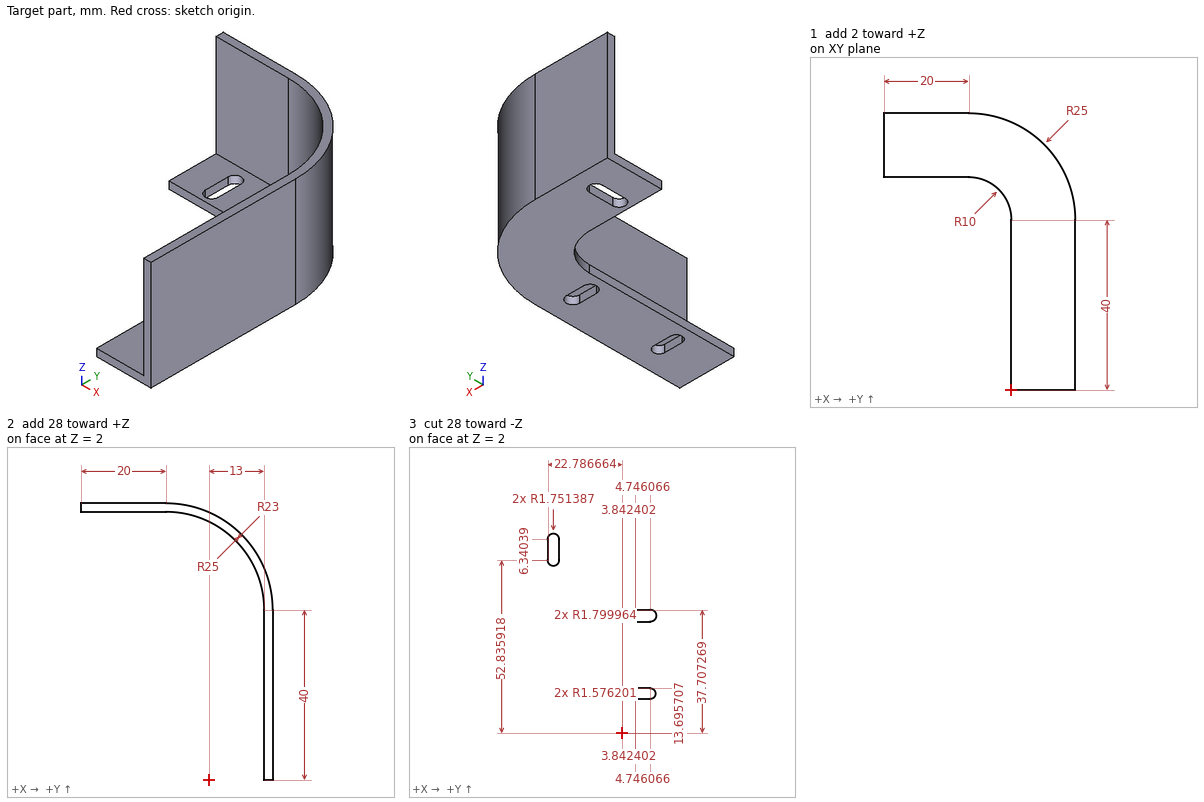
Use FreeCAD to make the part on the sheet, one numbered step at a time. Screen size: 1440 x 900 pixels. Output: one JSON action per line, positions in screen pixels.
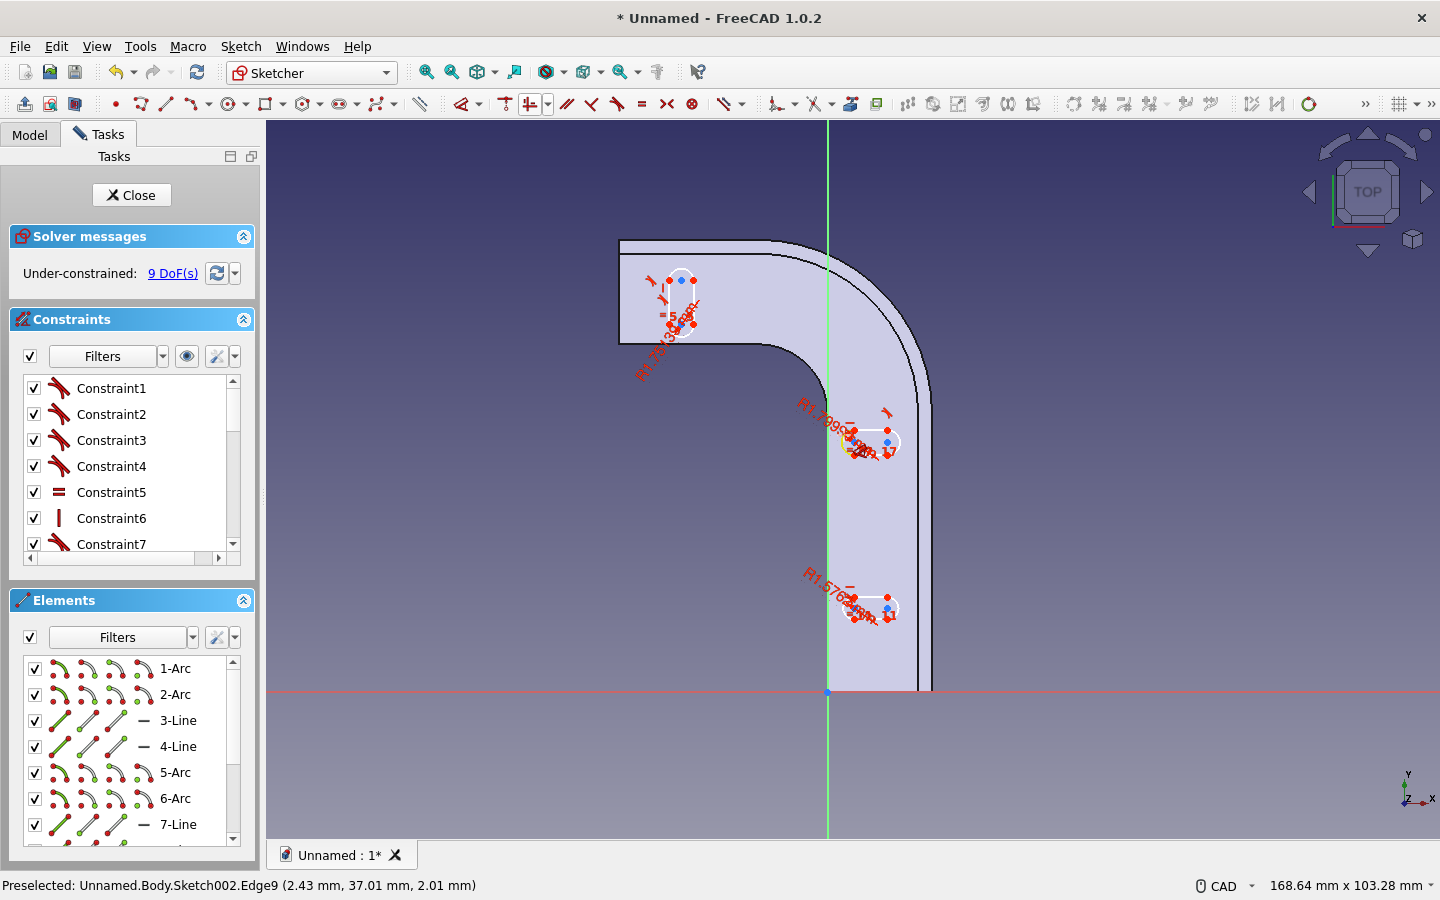
{"action": "left_click", "coordinate": [669, 312]}
{"action": "left_click", "coordinate": [635, 303]}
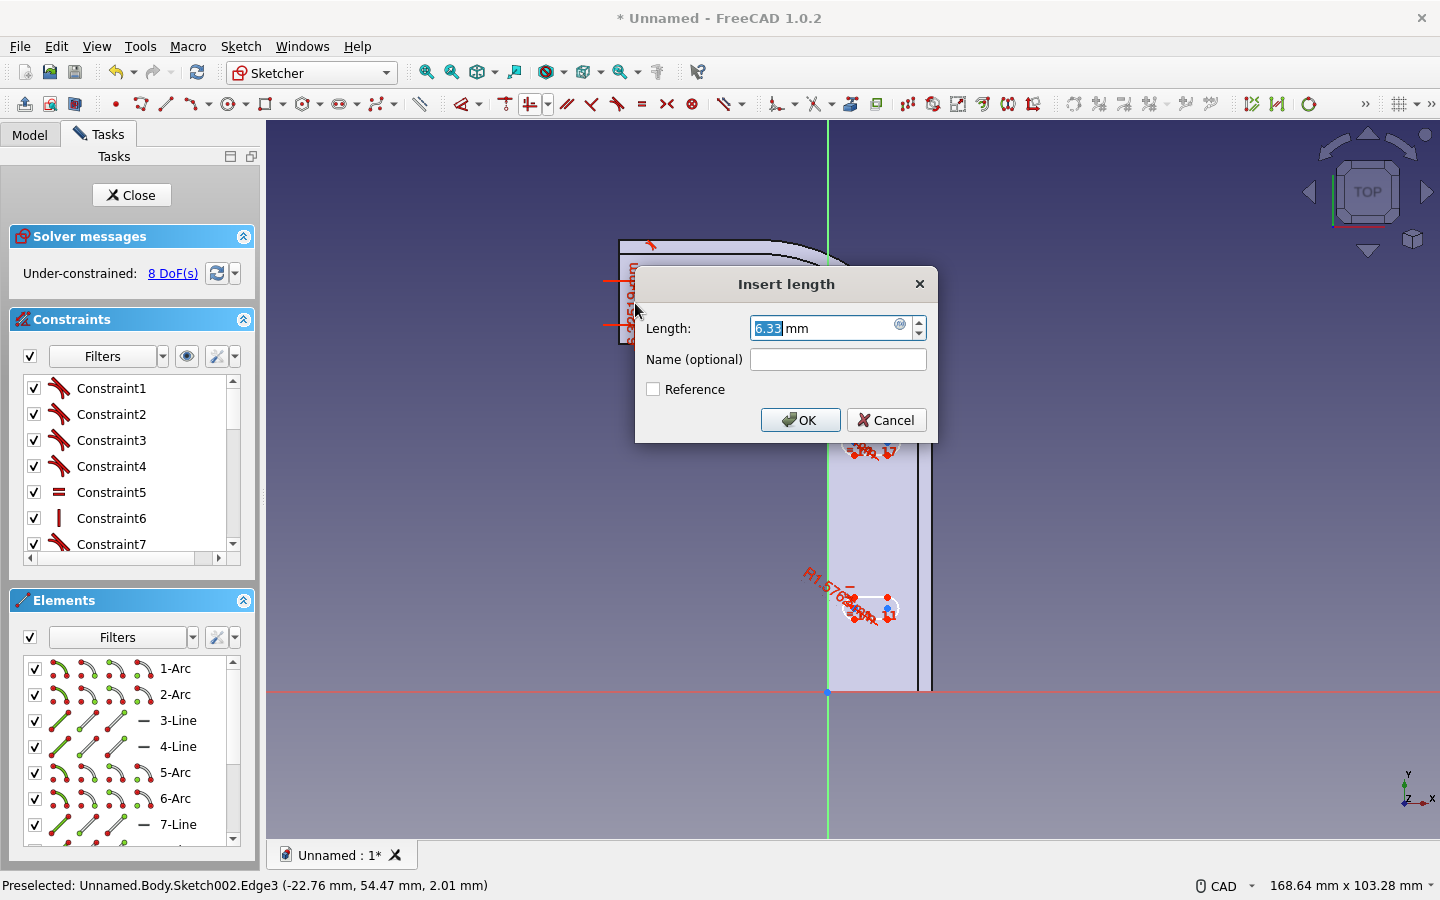
{"action": "type", "text": "6.34039"}
{"action": "key", "text": "Return"}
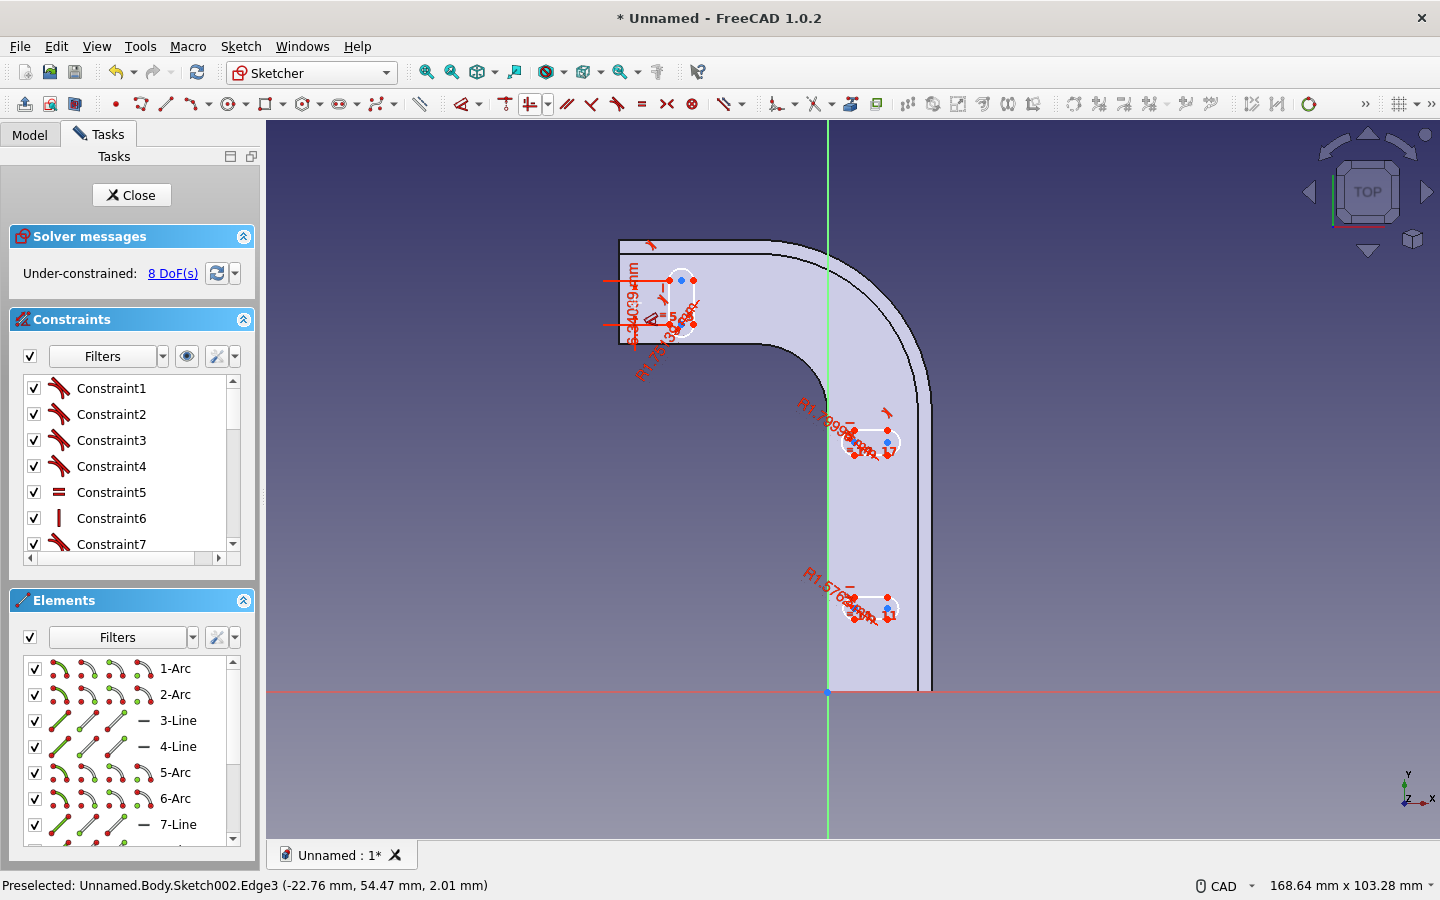
{"action": "scroll", "coordinate": [864, 597], "scroll_direction": "up", "scroll_amount": 2}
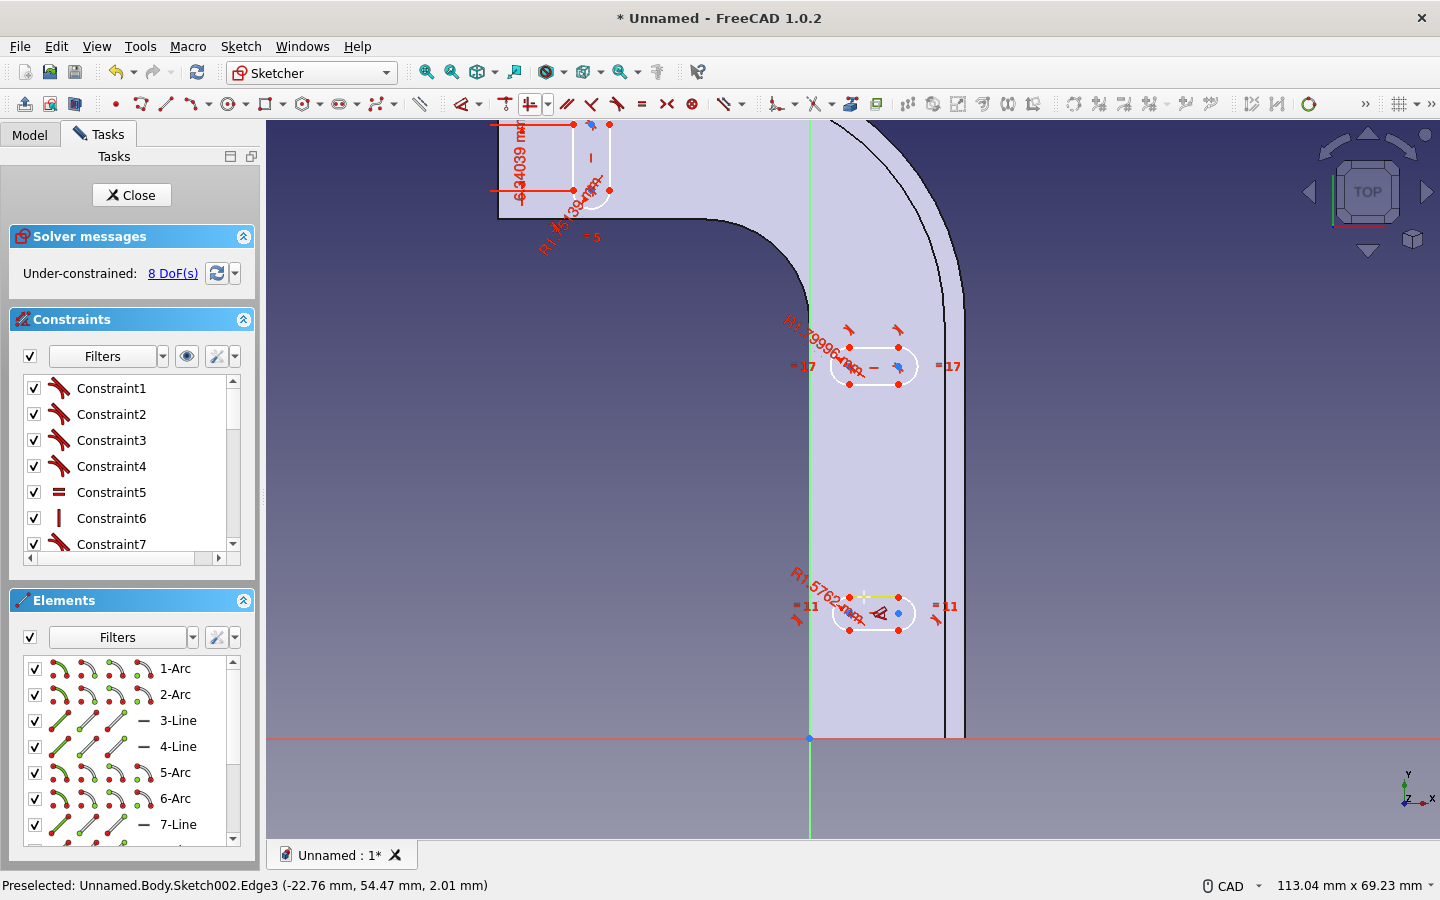
{"action": "left_click", "coordinate": [864, 597]}
{"action": "left_click", "coordinate": [874, 563]}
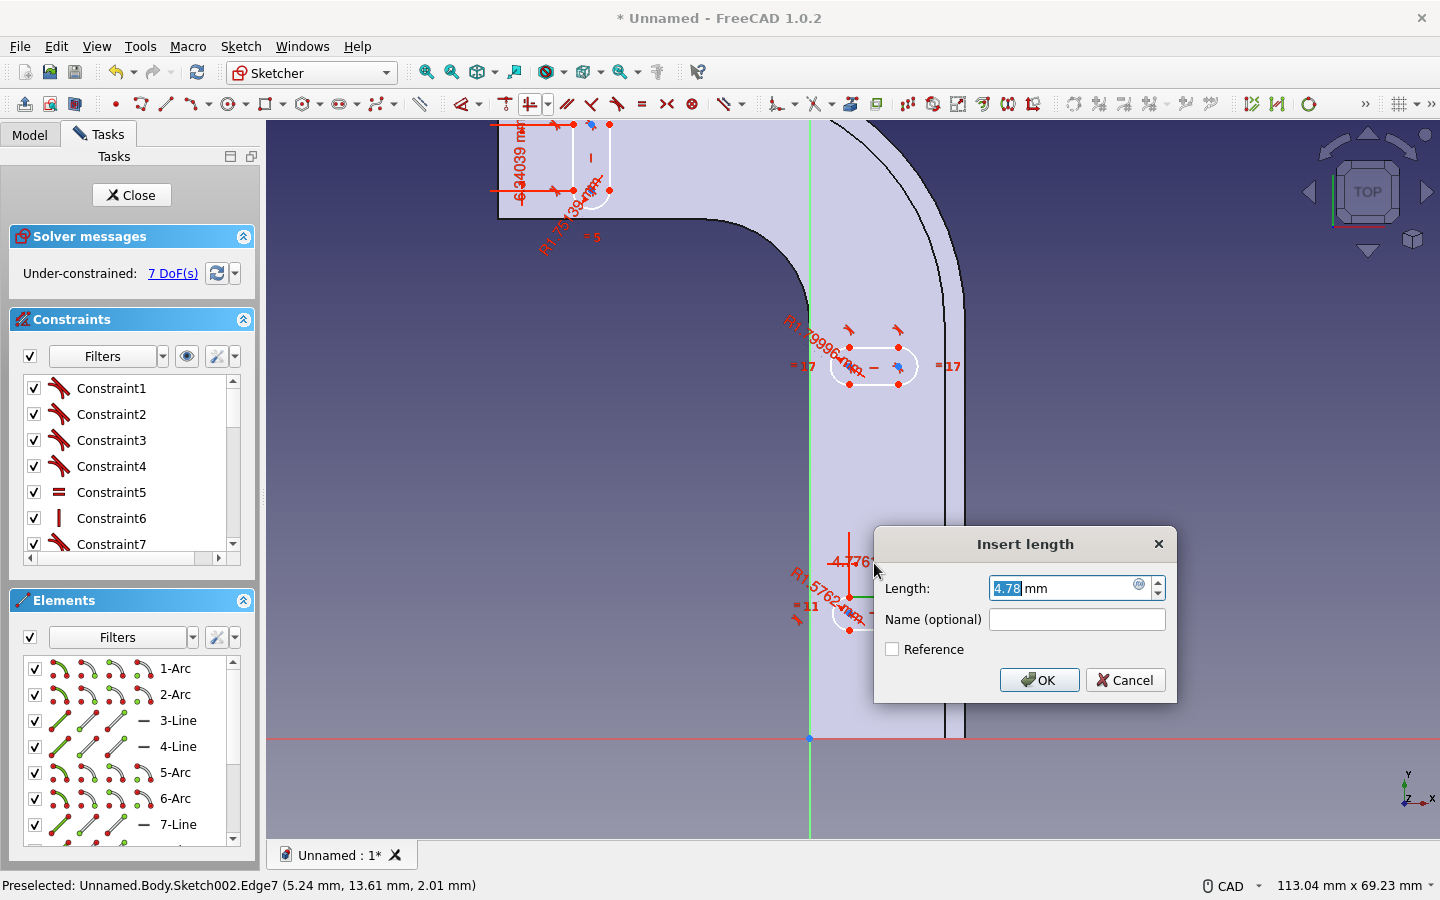
{"action": "type", "text": "4.746066"}
{"action": "key", "text": "Return"}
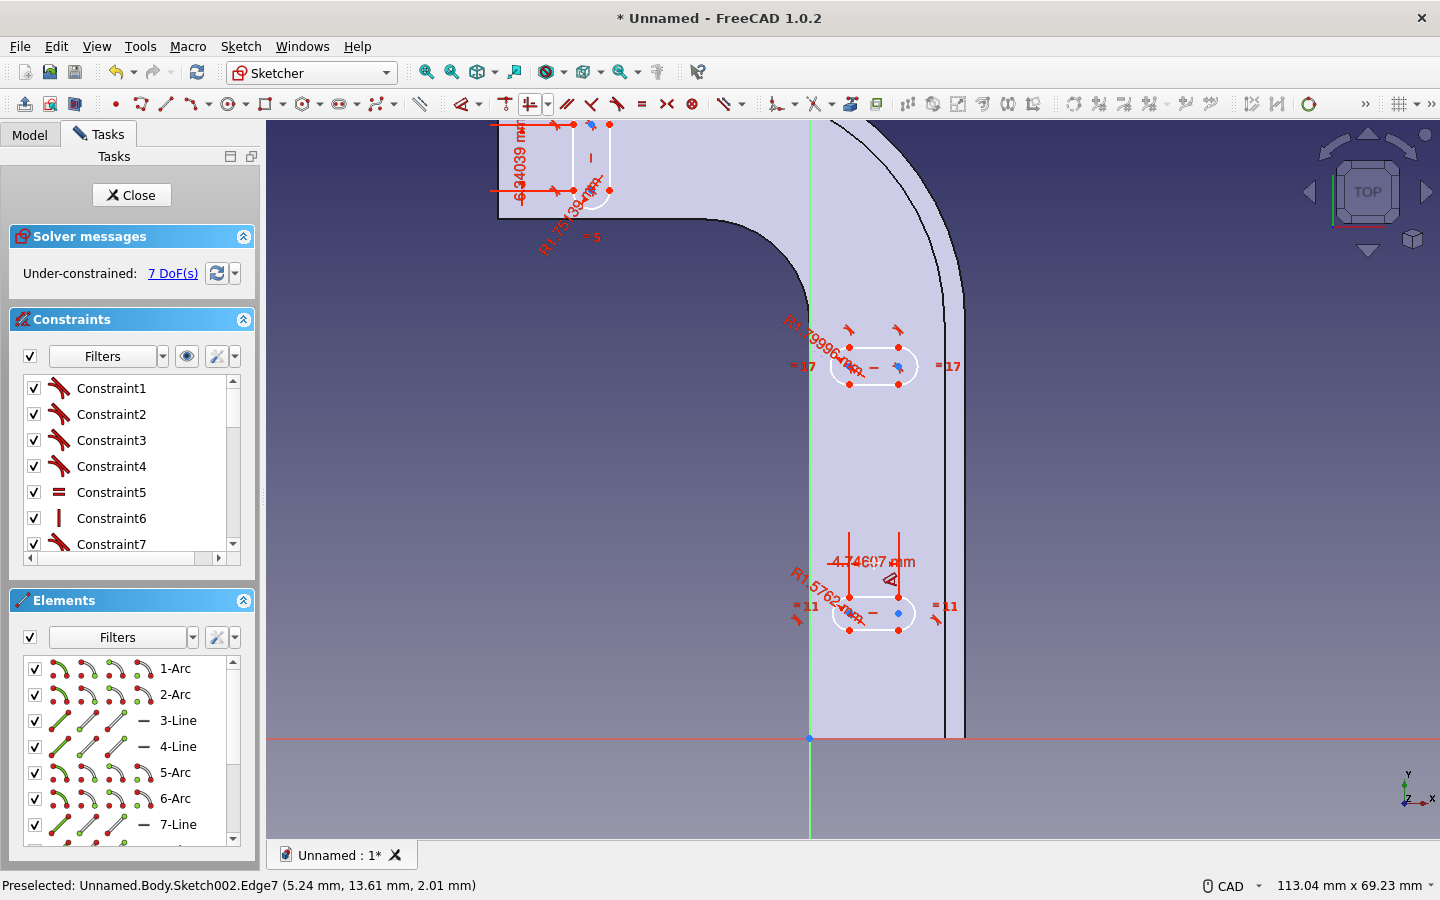
{"action": "left_click", "coordinate": [864, 348]}
{"action": "left_click", "coordinate": [874, 314]}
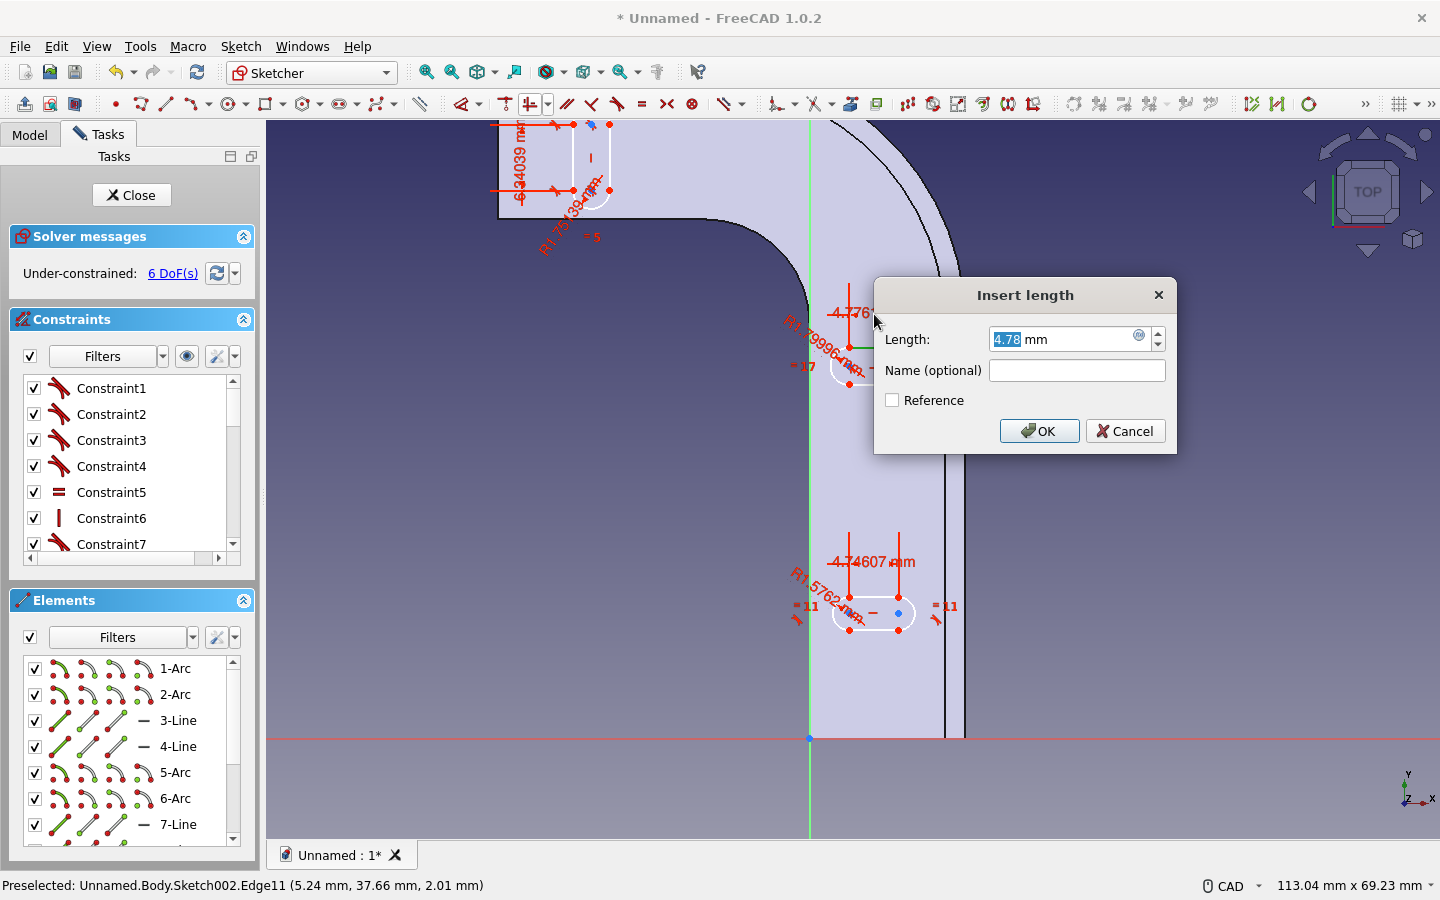
{"action": "type", "text": "4.746066"}
{"action": "key", "text": "Return"}